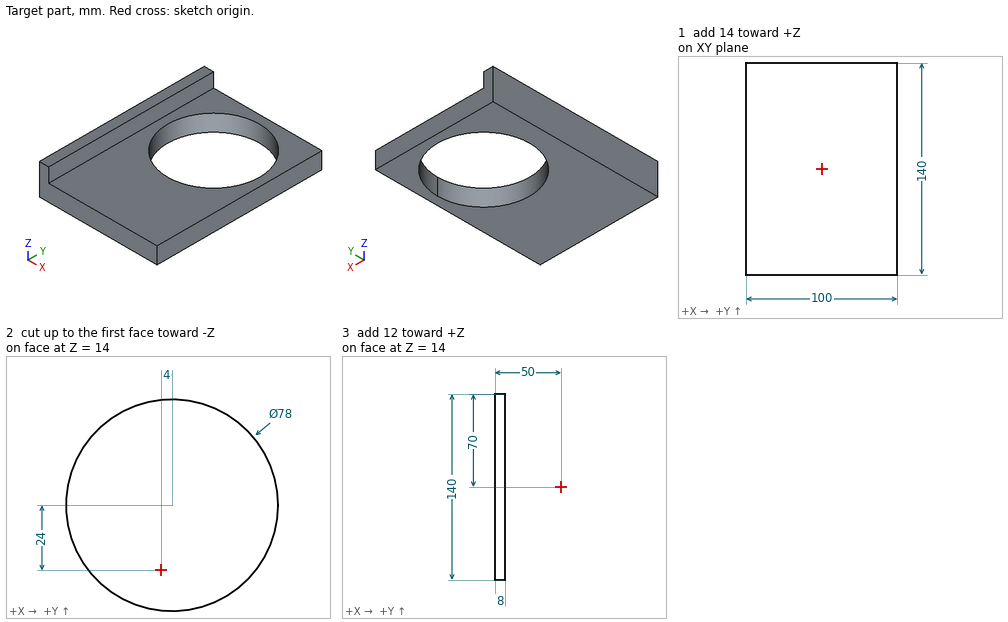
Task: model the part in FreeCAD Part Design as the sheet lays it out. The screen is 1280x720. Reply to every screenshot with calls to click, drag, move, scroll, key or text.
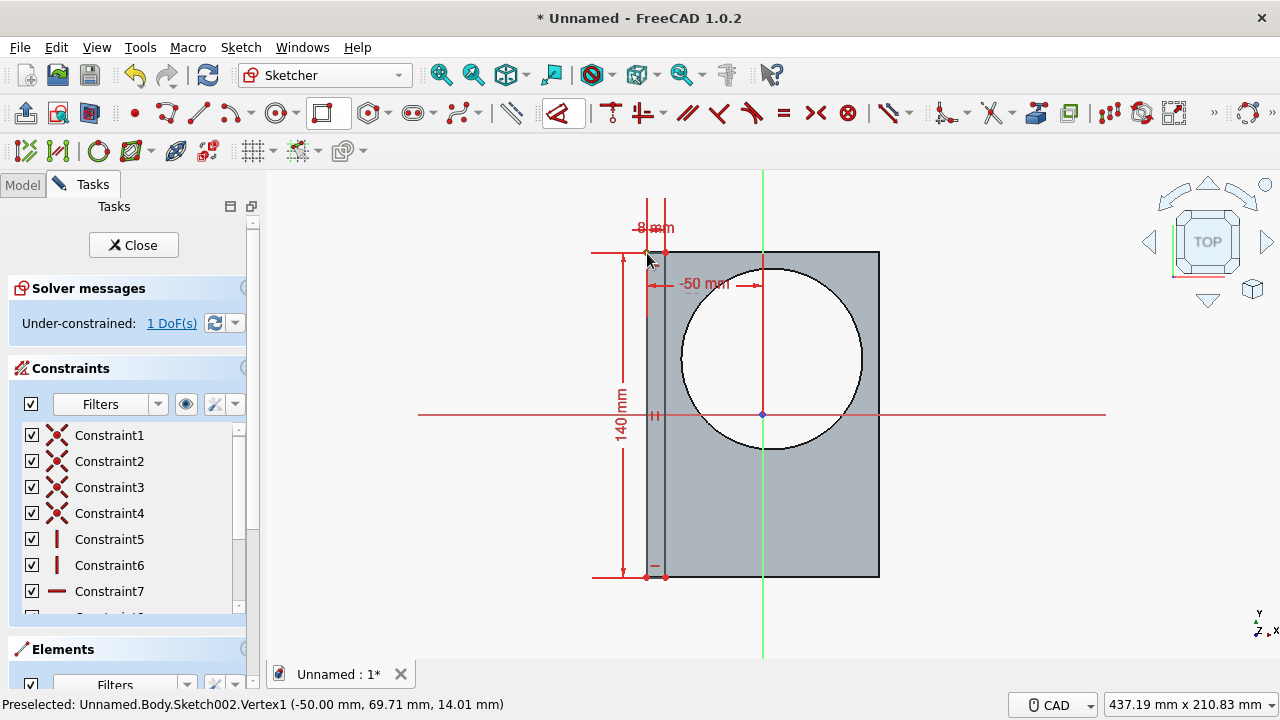
key(i)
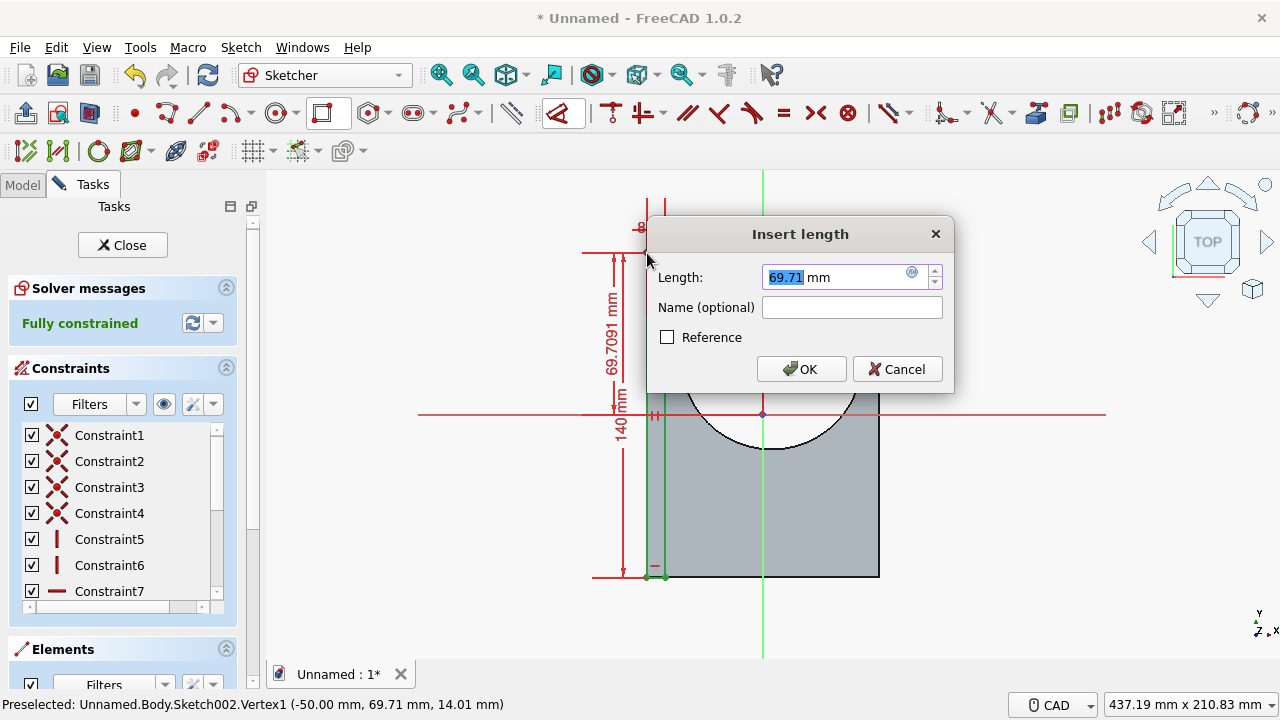
text(70)
key(Return)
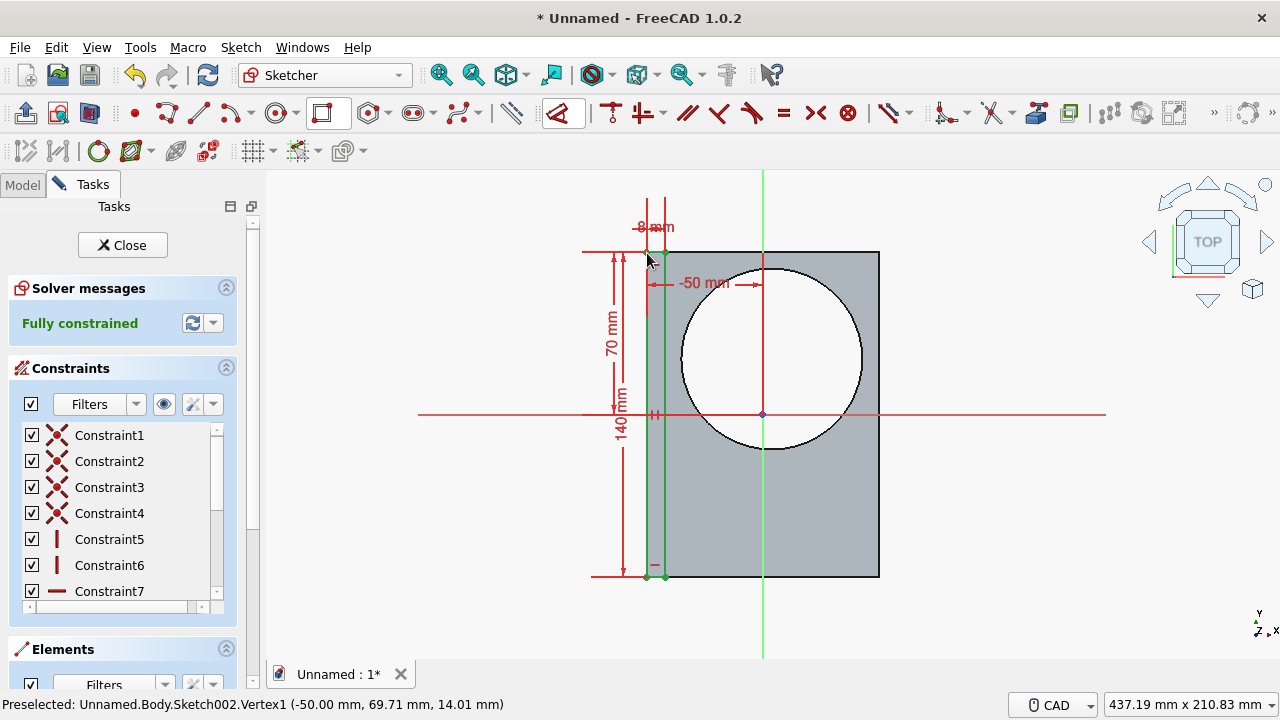
click(123, 245)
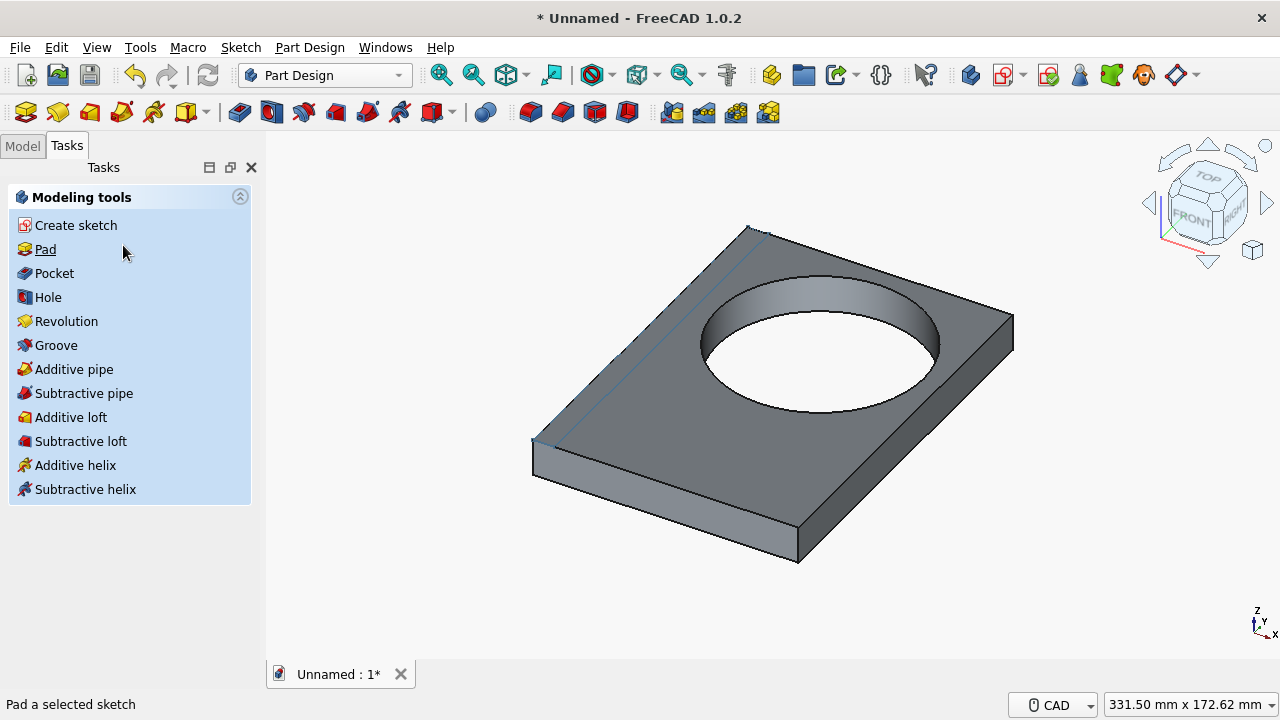
click(26, 112)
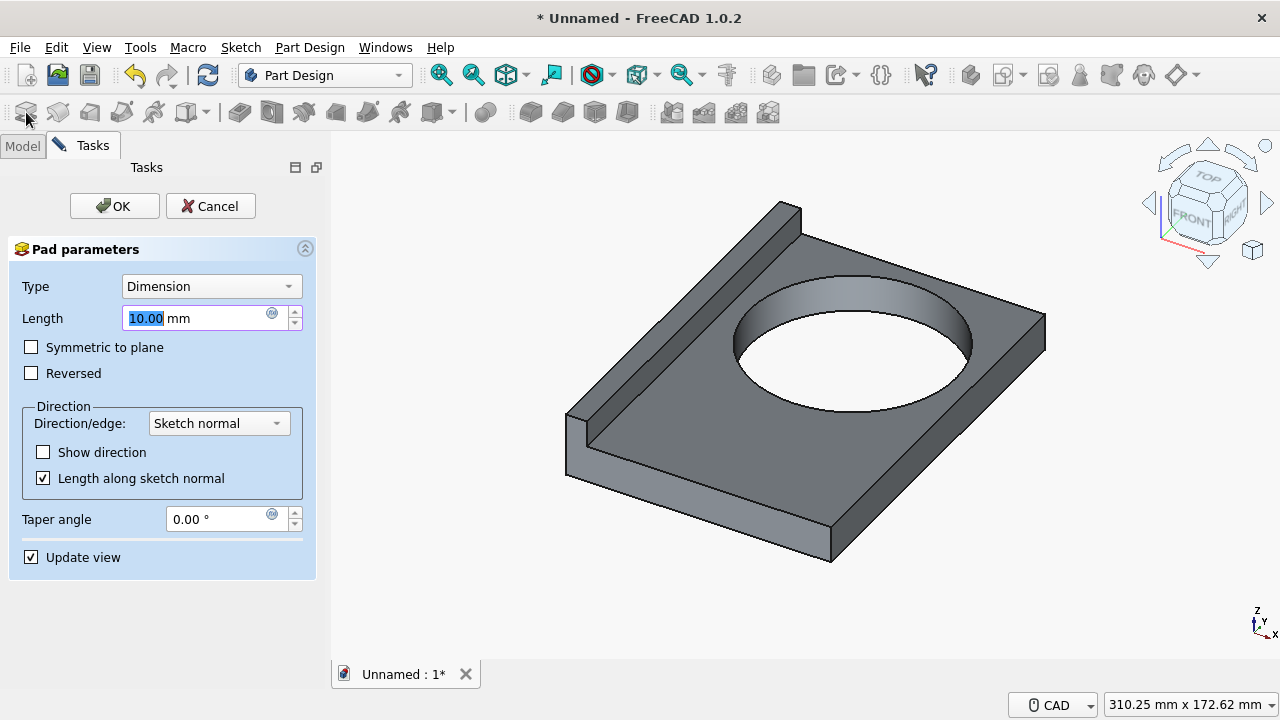
text(12)
key(Tab)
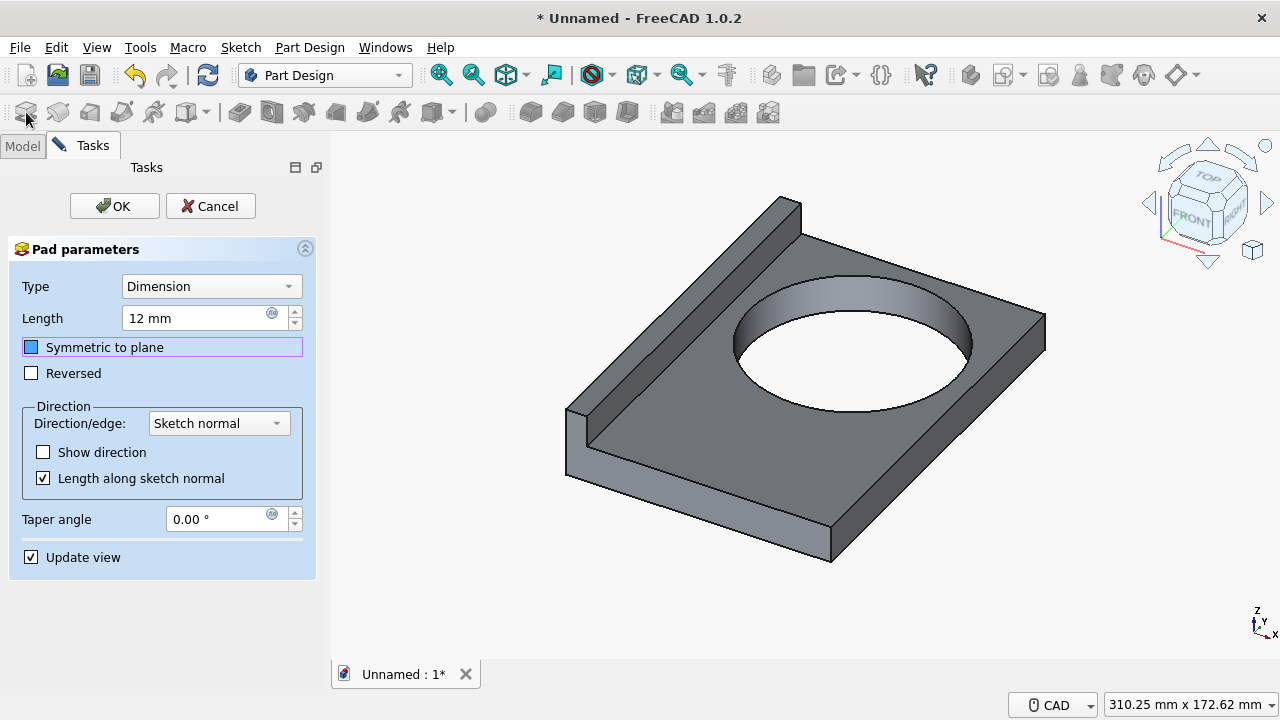
click(115, 206)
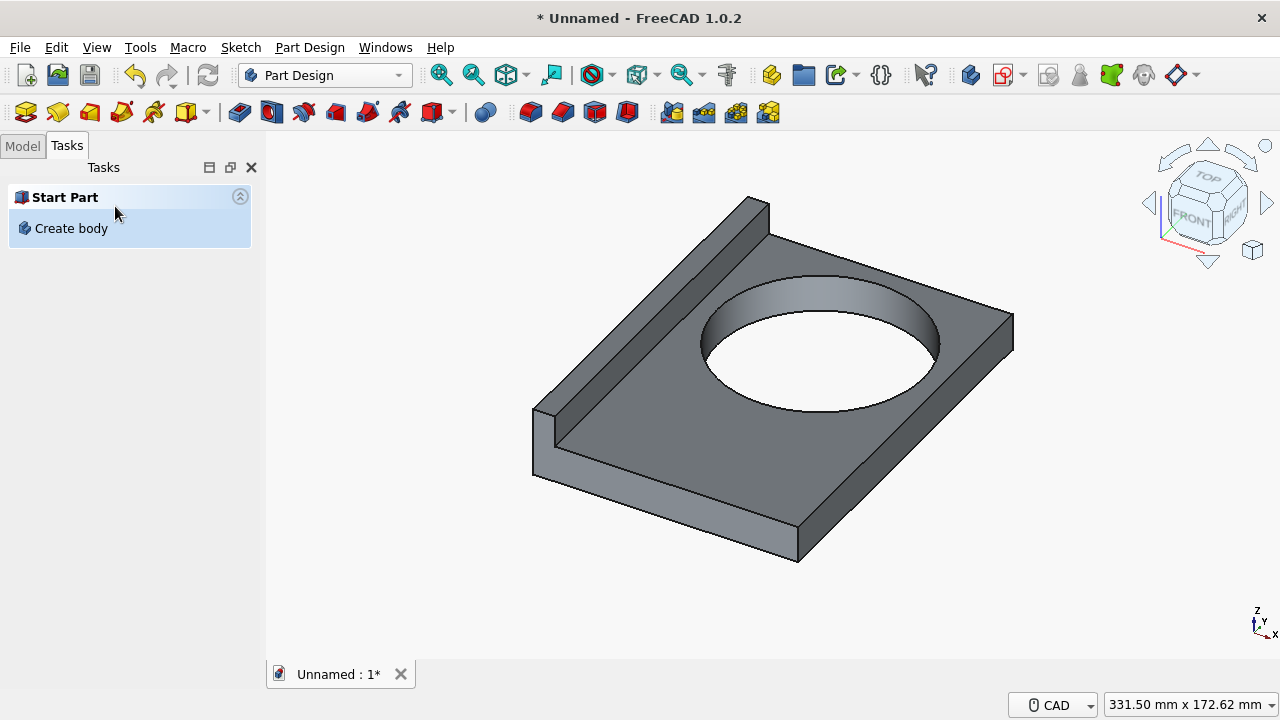
key(0)